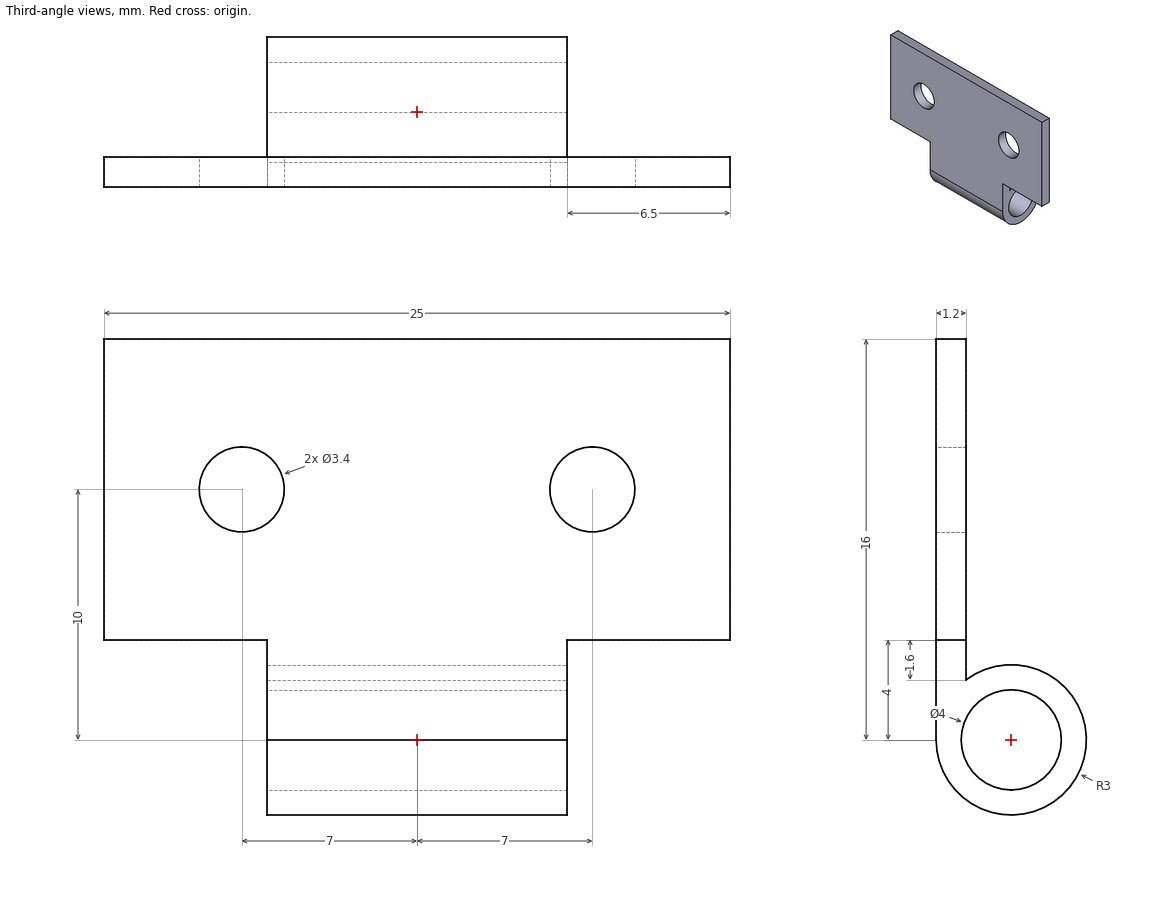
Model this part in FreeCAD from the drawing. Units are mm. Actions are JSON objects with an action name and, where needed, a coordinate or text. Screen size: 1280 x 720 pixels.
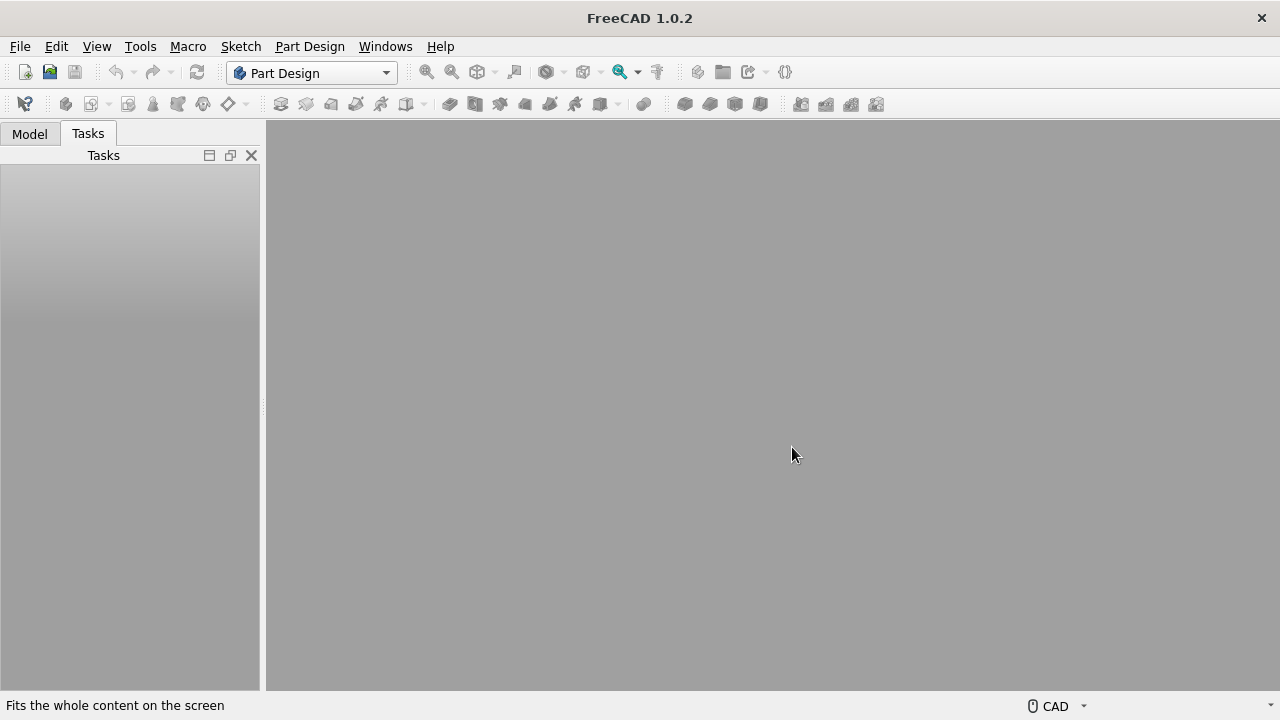
{"action": "left_click", "coordinate": [25, 72]}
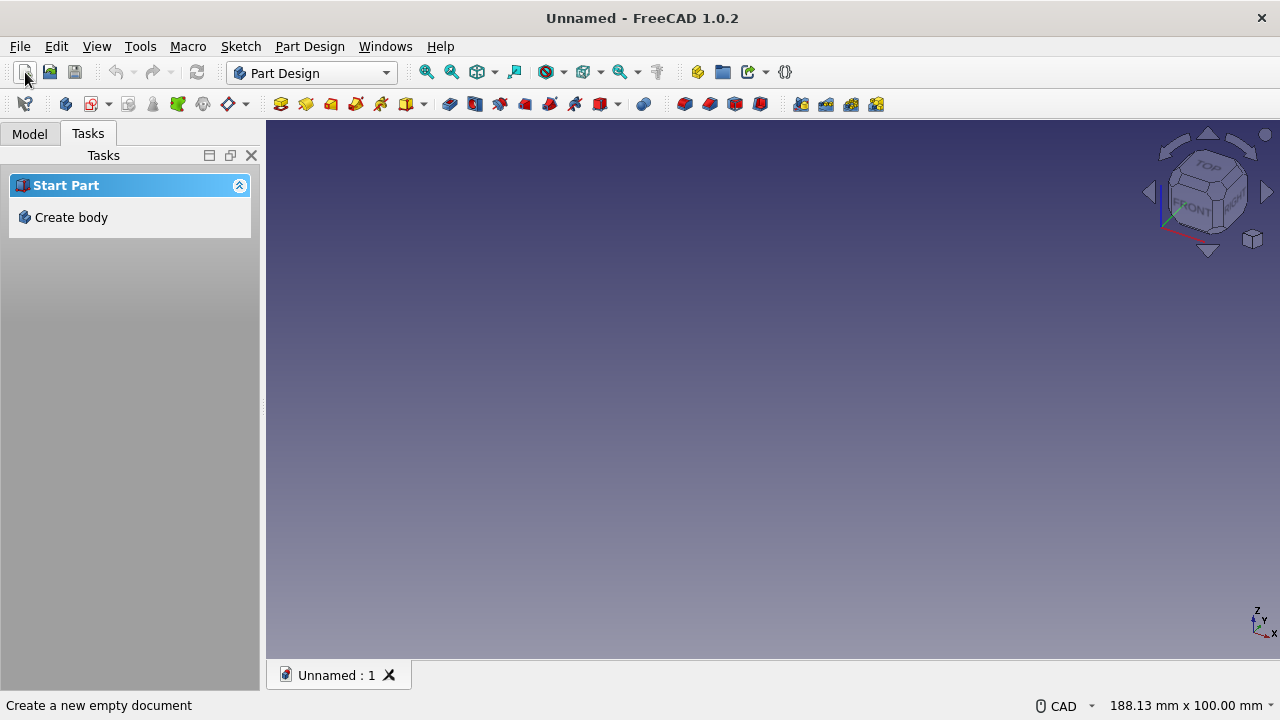
{"action": "left_click", "coordinate": [90, 104]}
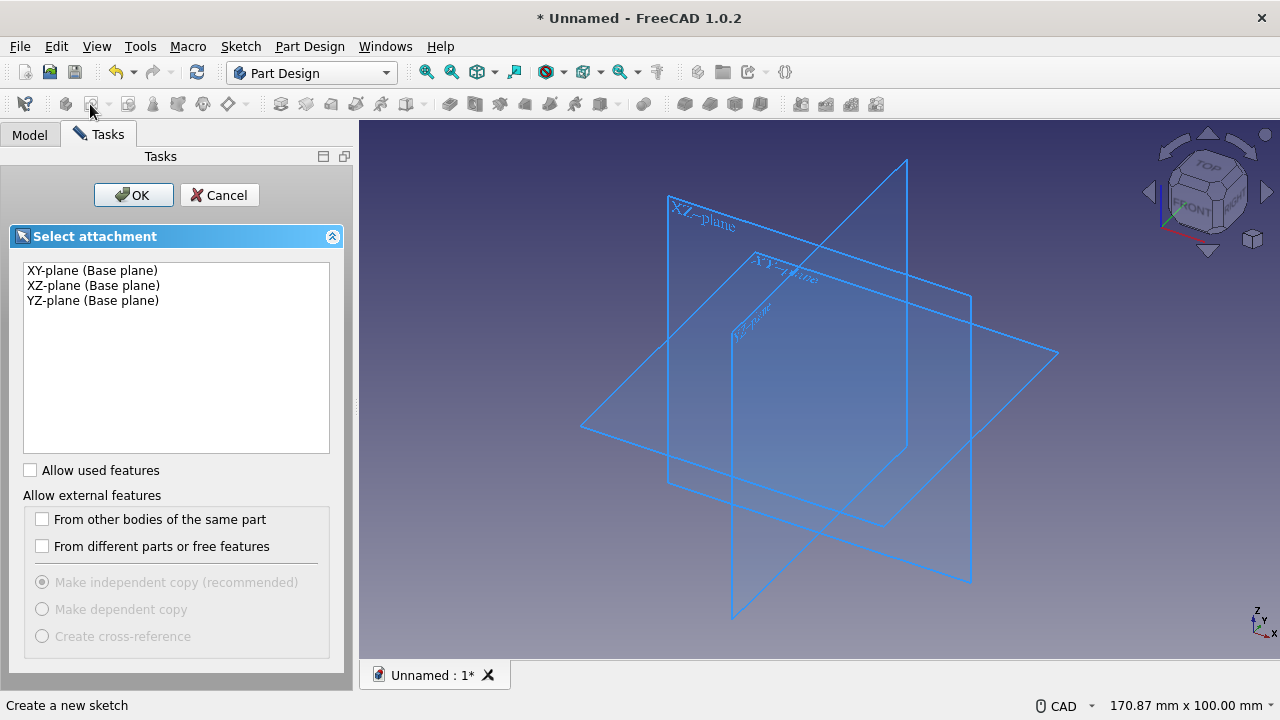
{"action": "left_click", "coordinate": [84, 300]}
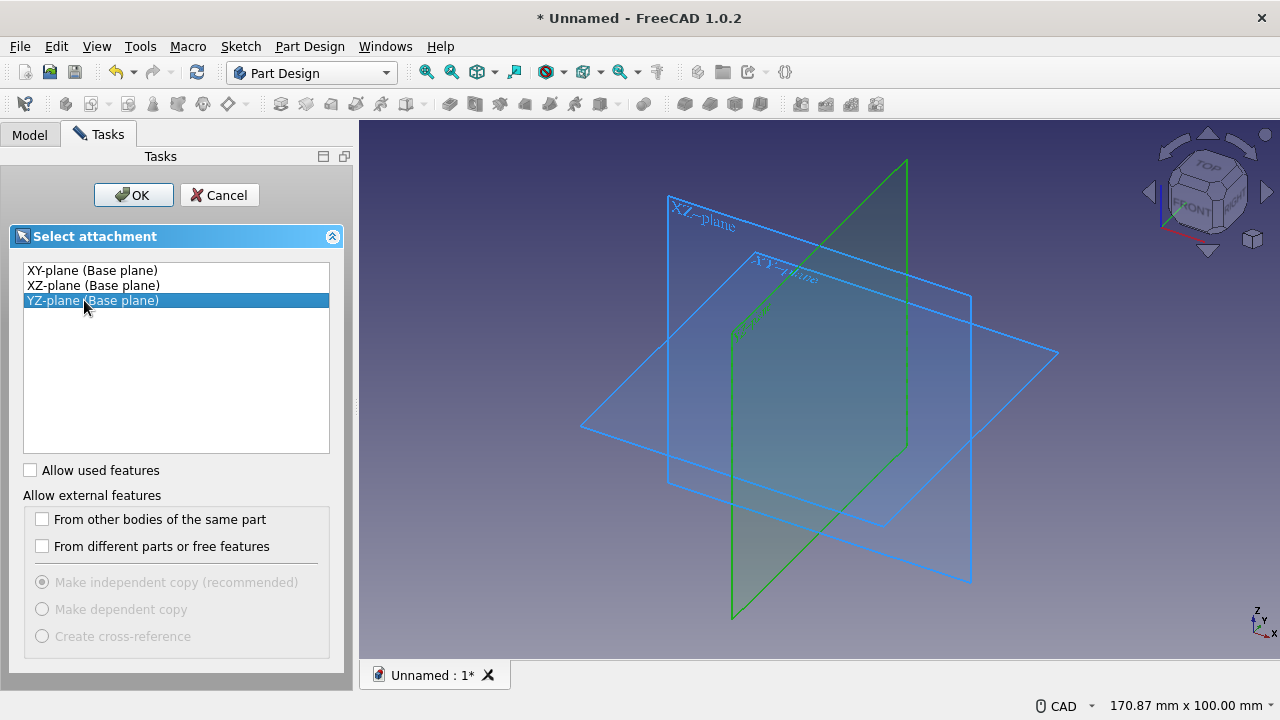
{"action": "left_click", "coordinate": [134, 195]}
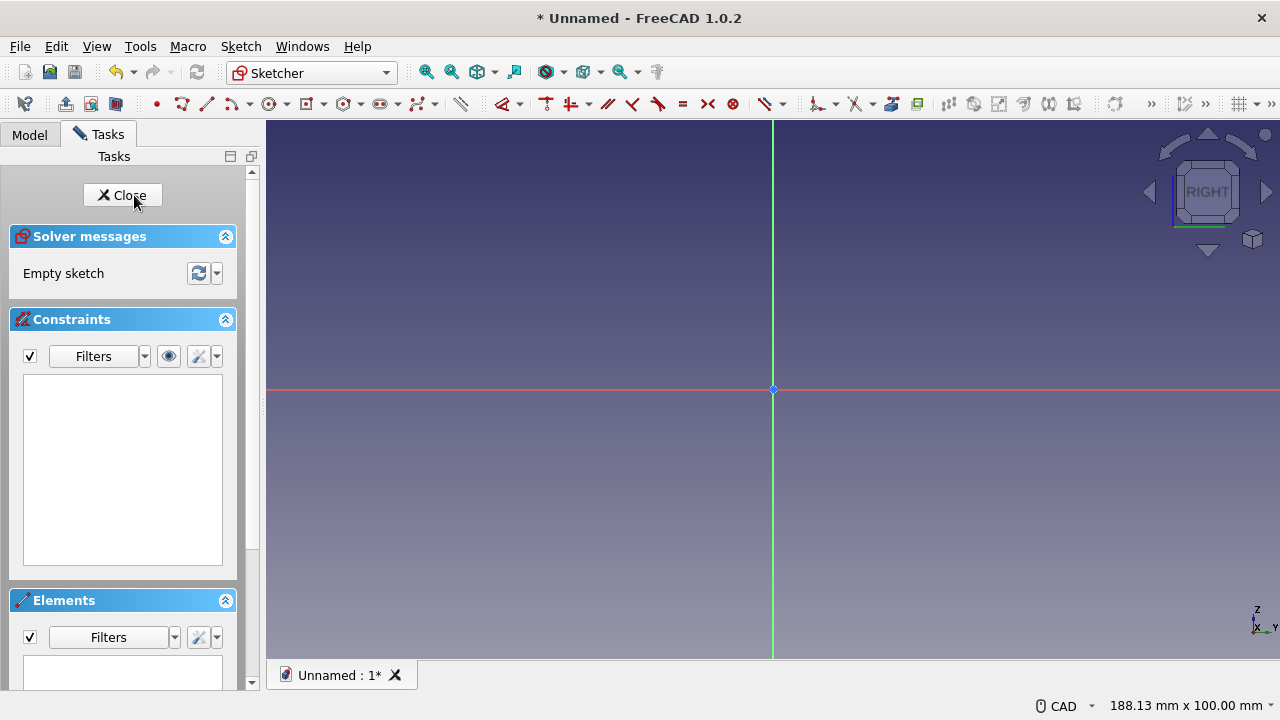
{"action": "scroll", "coordinate": [801, 336], "scroll_direction": "up", "scroll_amount": 6}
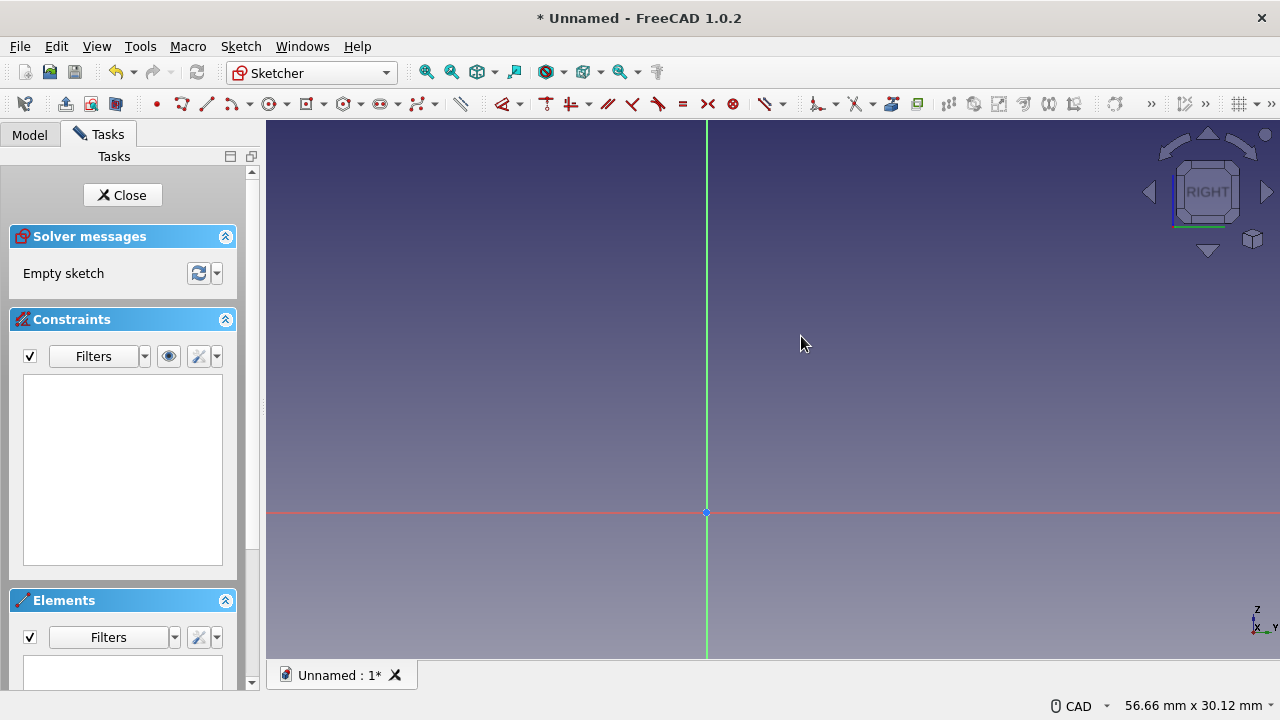
{"action": "left_click", "coordinate": [182, 104]}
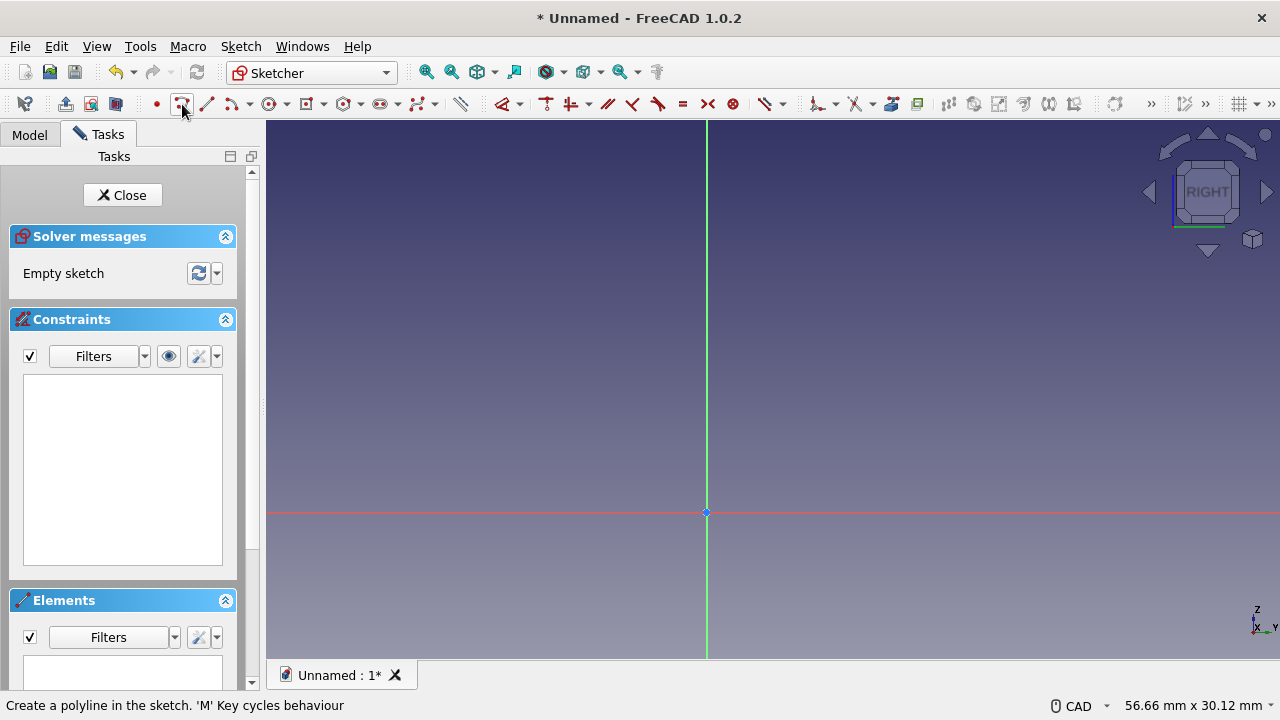
{"action": "left_click", "coordinate": [675, 470]}
{"action": "left_click", "coordinate": [675, 226]}
{"action": "left_click", "coordinate": [653, 226]}
{"action": "left_click", "coordinate": [653, 513]}
{"action": "right_click", "coordinate": [653, 513]}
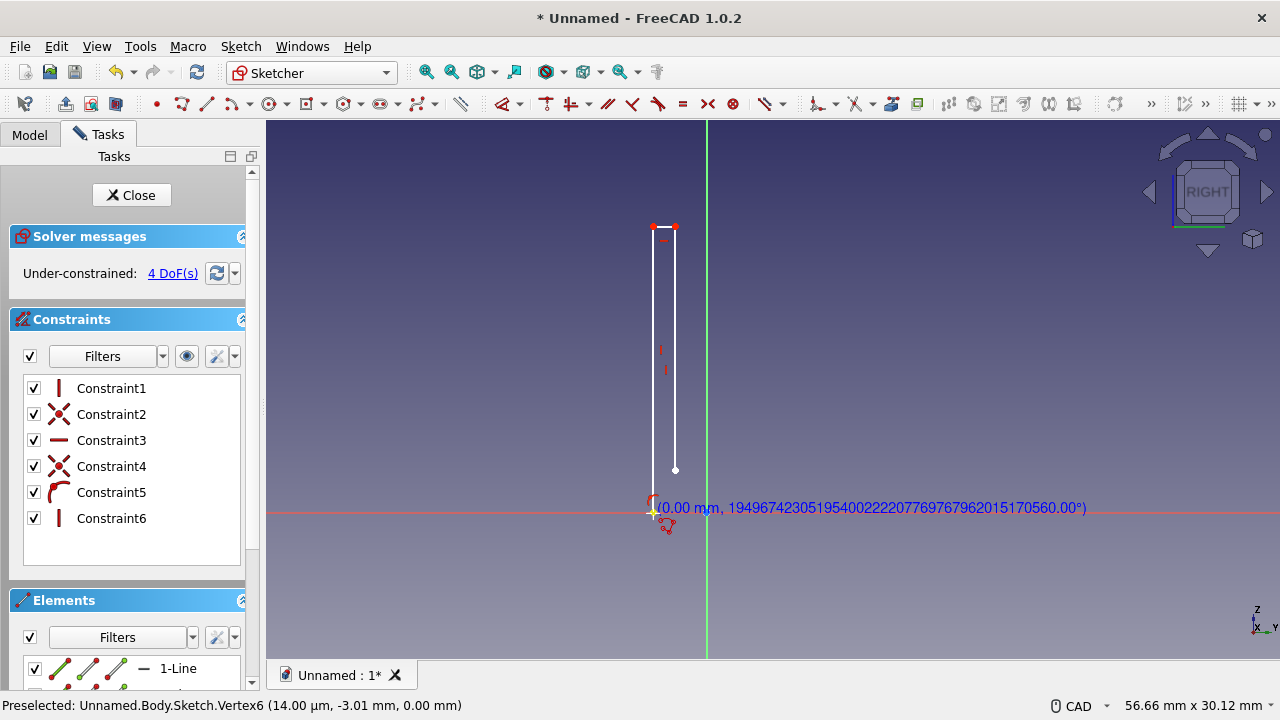
{"action": "key", "text": "g 3 a"}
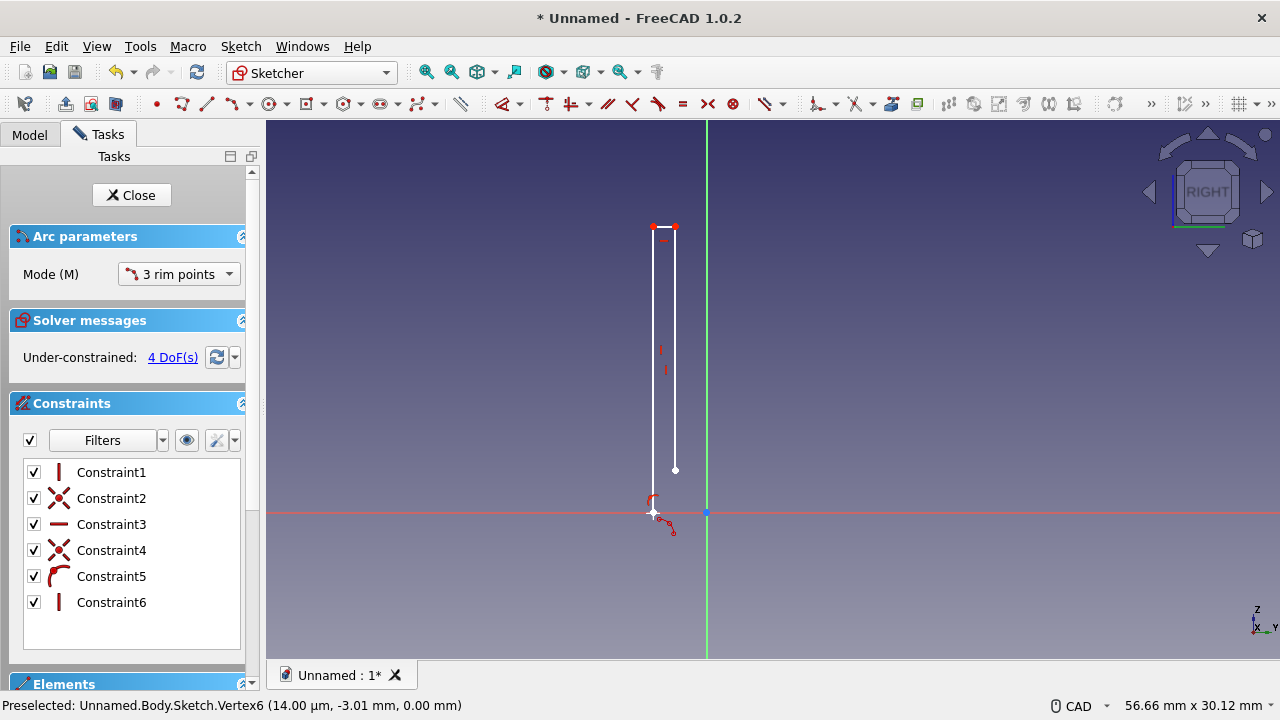
{"action": "left_click", "coordinate": [653, 513]}
{"action": "left_click", "coordinate": [675, 471]}
{"action": "left_click", "coordinate": [755, 537]}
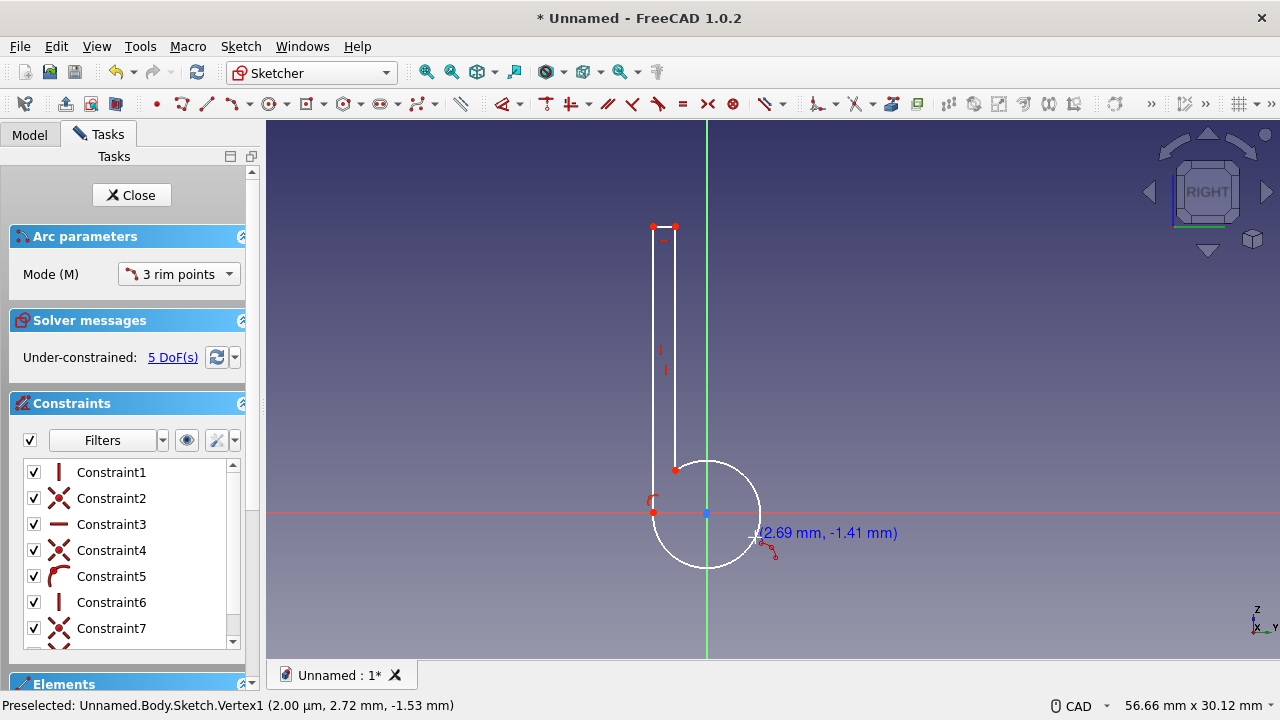
{"action": "left_click", "coordinate": [268, 104]}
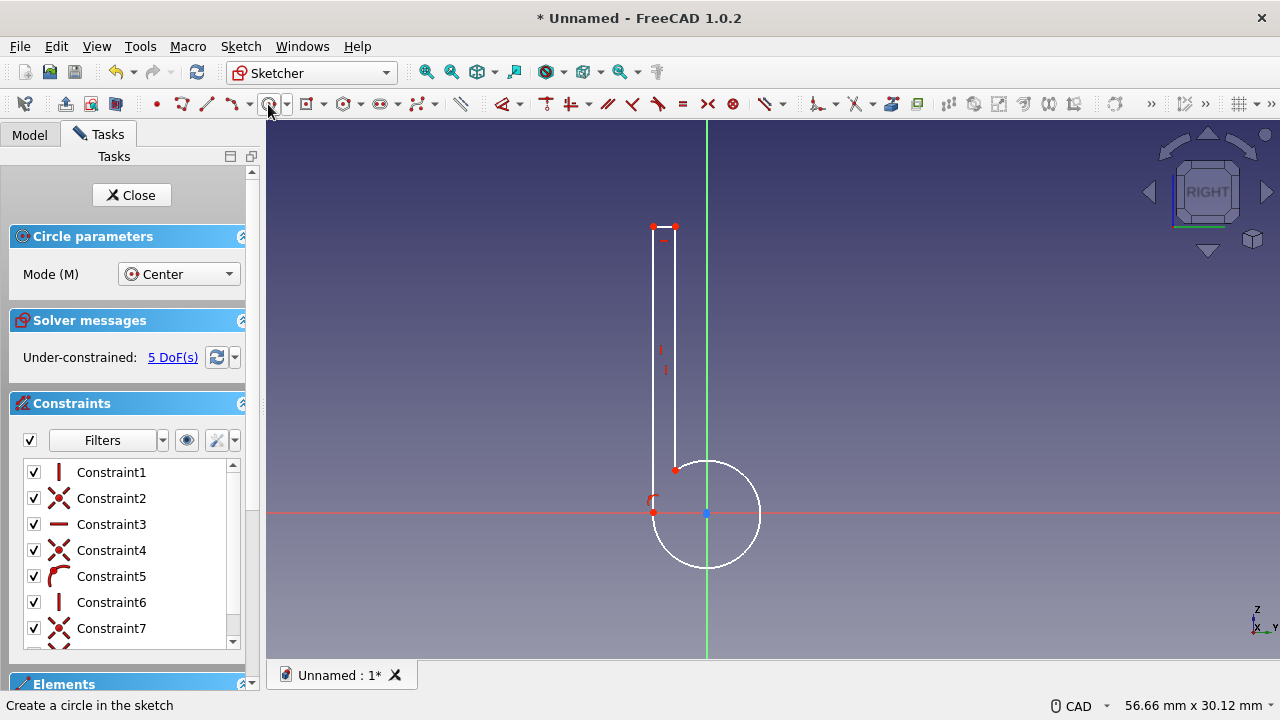
{"action": "left_click", "coordinate": [707, 513]}
{"action": "mouse_move", "coordinate": [732, 487]}